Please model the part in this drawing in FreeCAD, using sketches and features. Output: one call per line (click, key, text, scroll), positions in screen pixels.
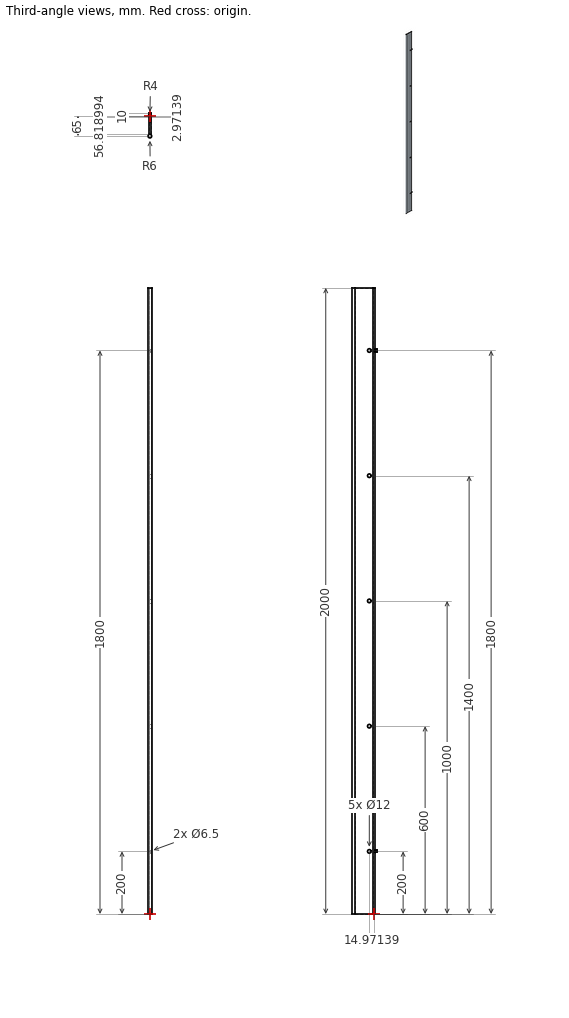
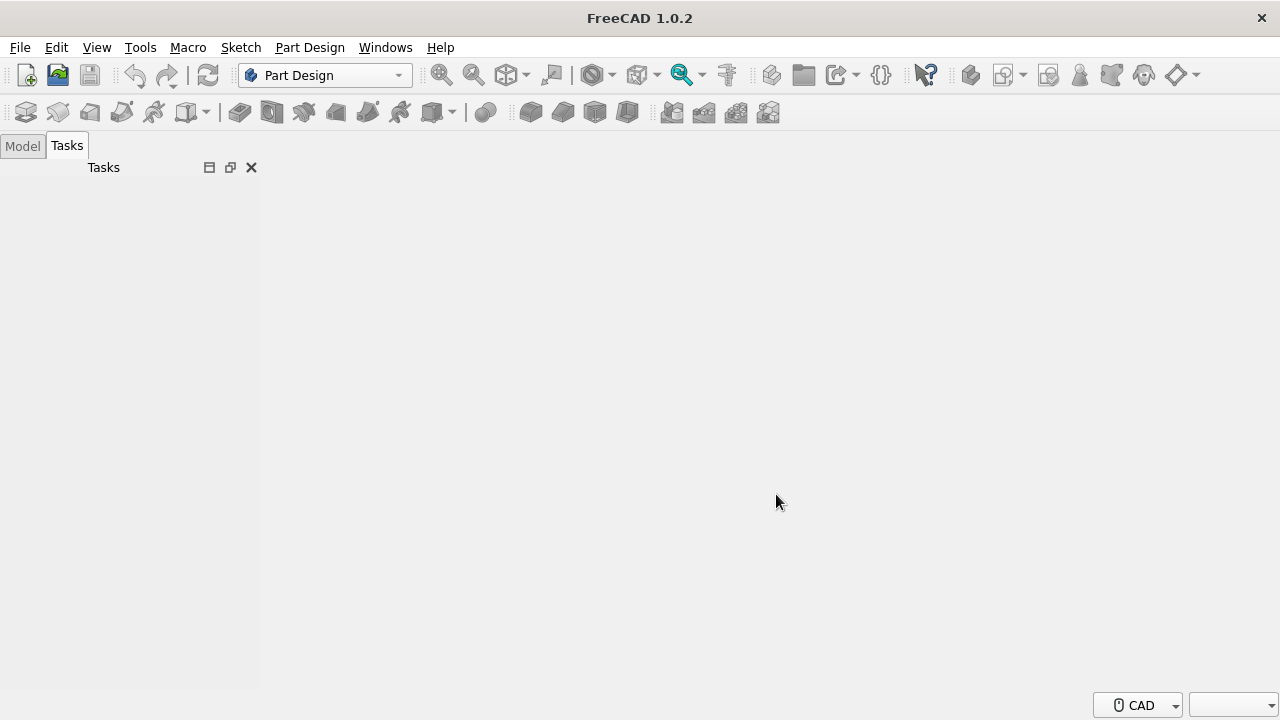
key(ctrl+n)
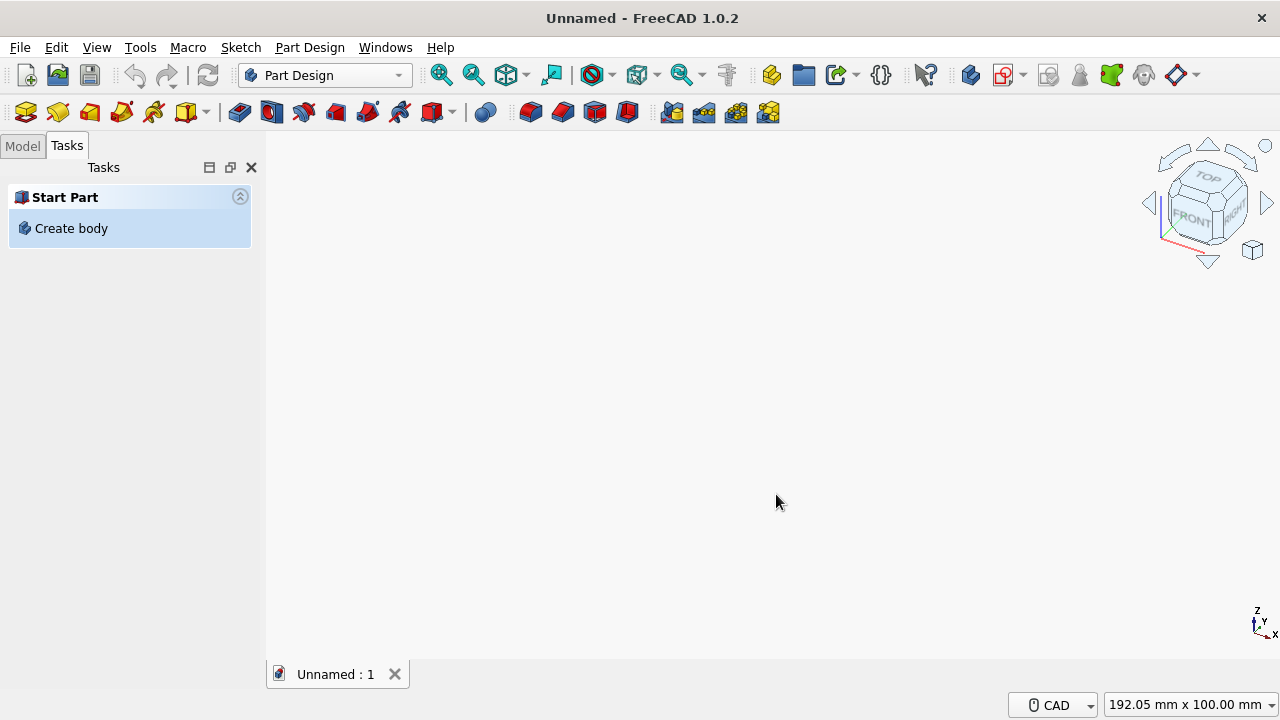
click(1004, 76)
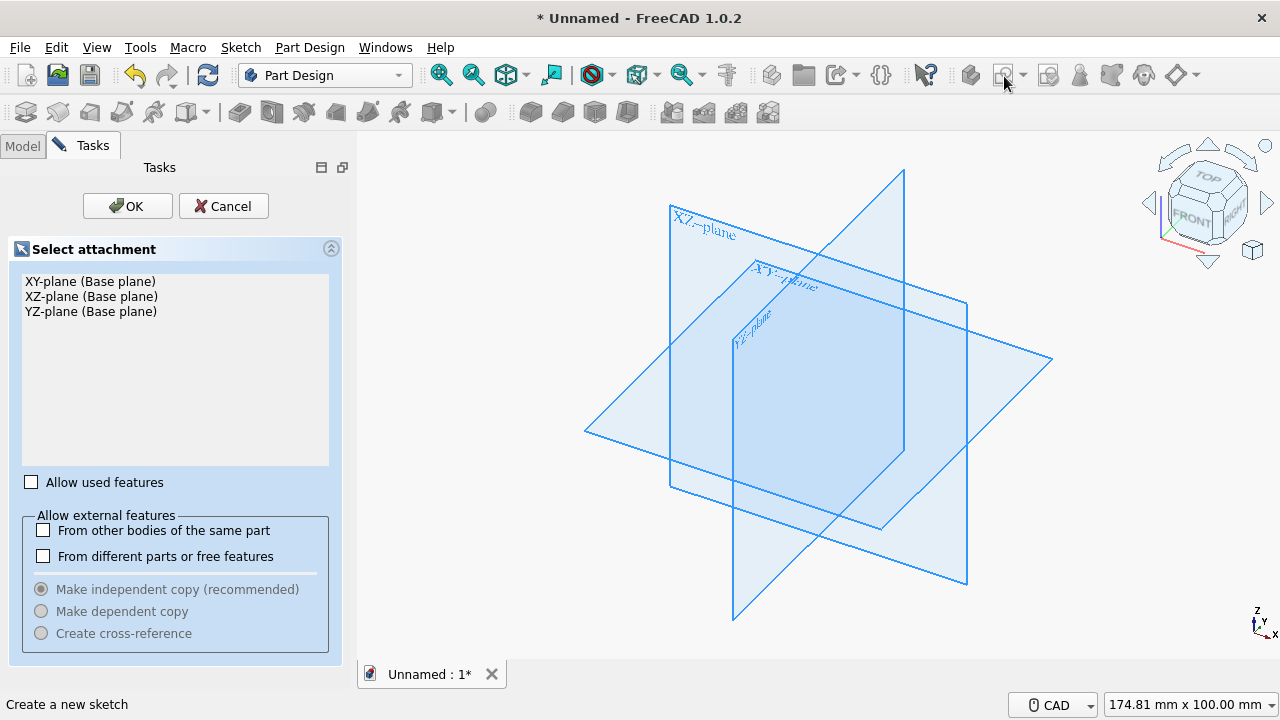
click(82, 282)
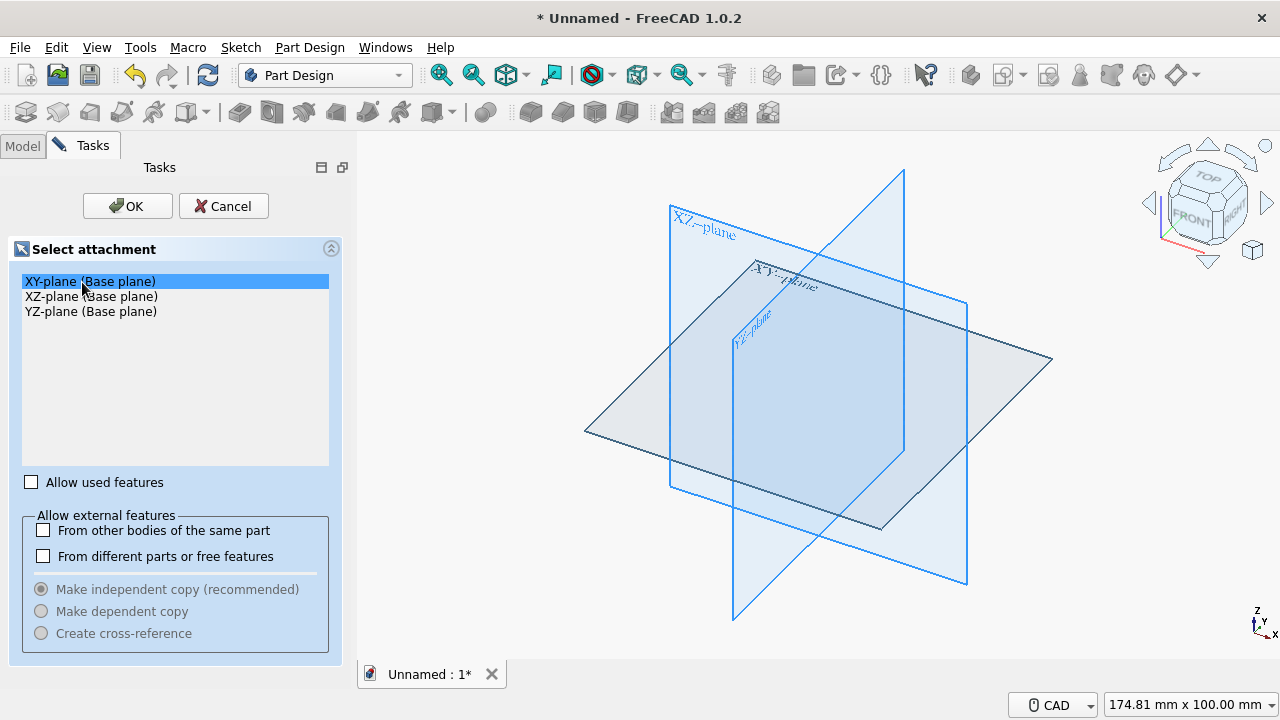
click(128, 206)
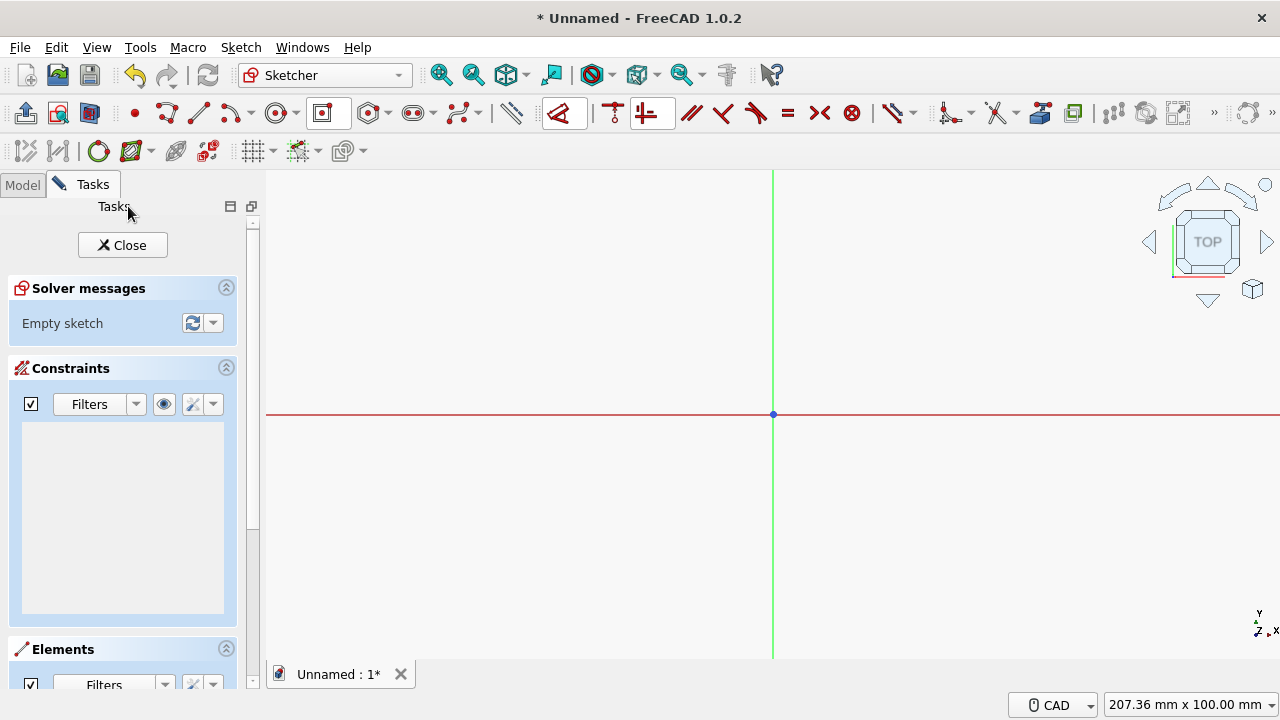
scroll(566, 198, down, 2)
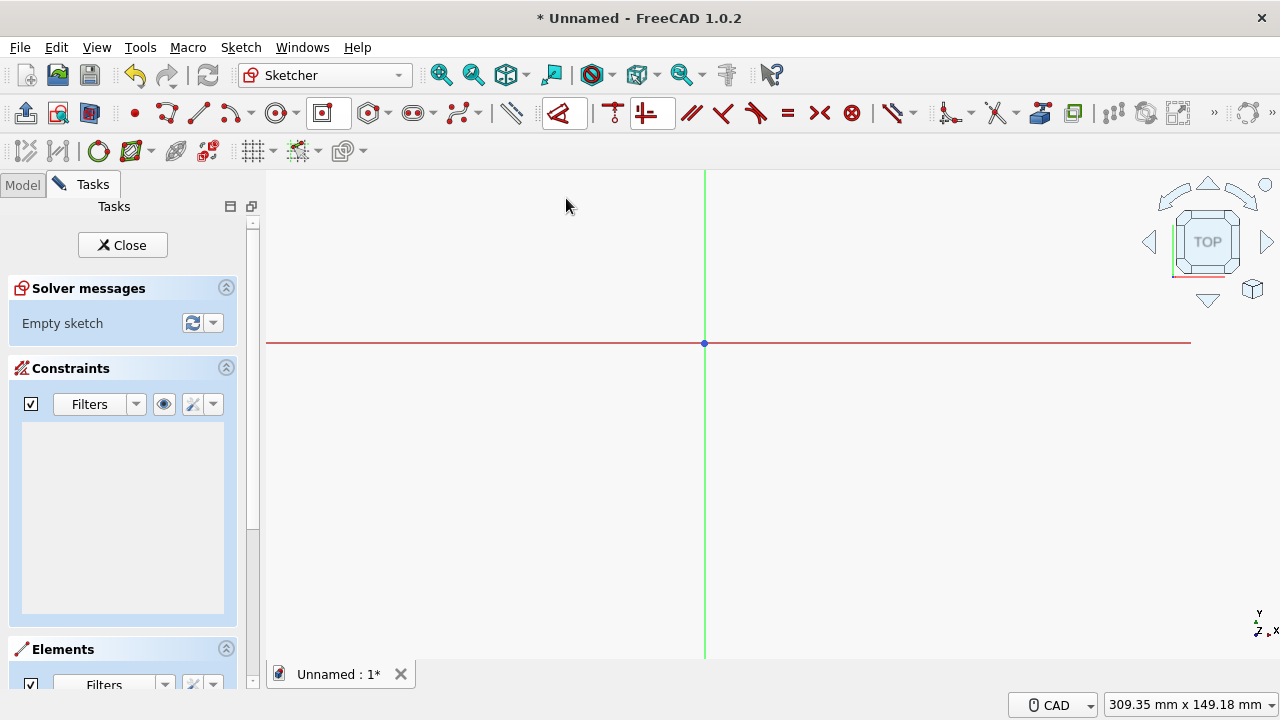
key(g)
key(l)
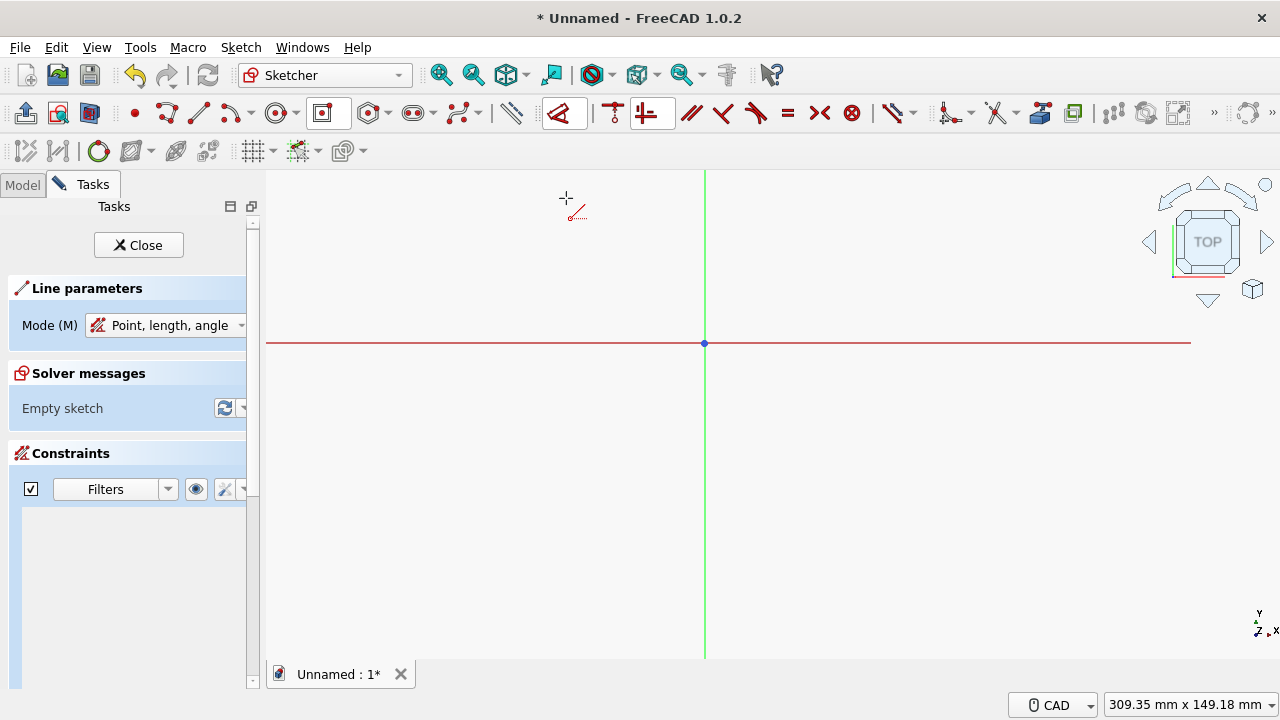
scroll(696, 353, up, 3)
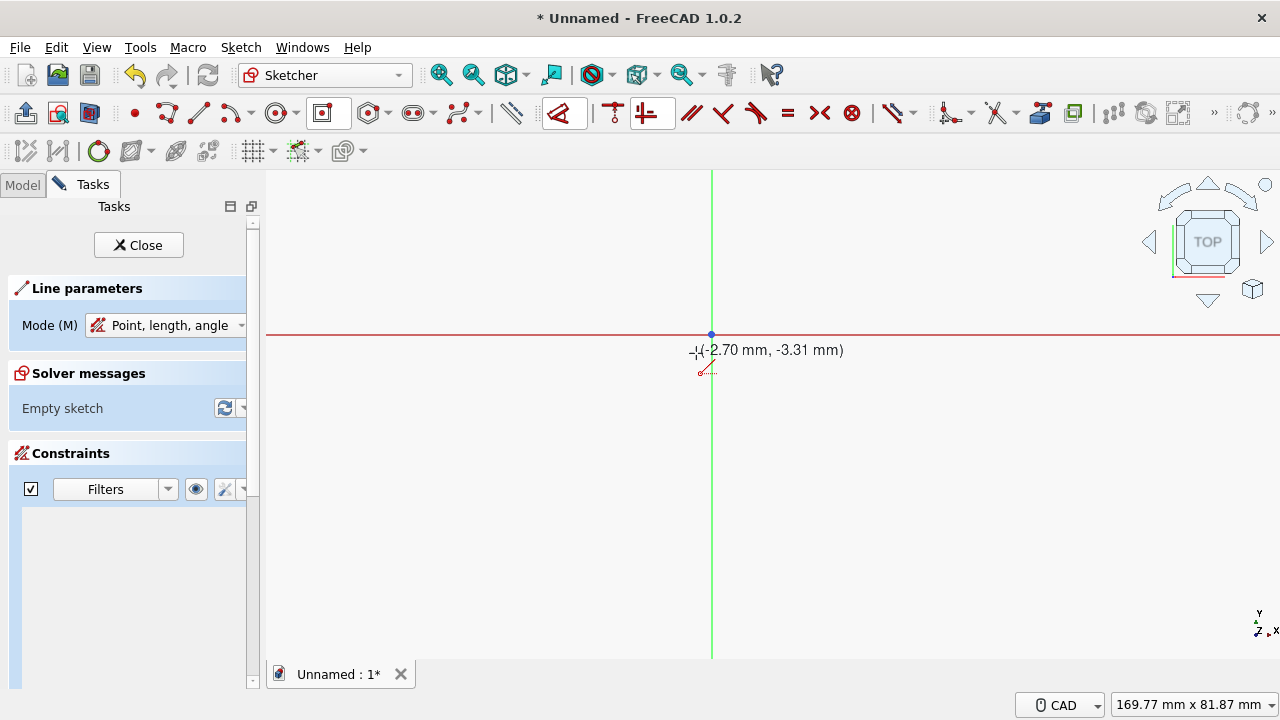
click(695, 352)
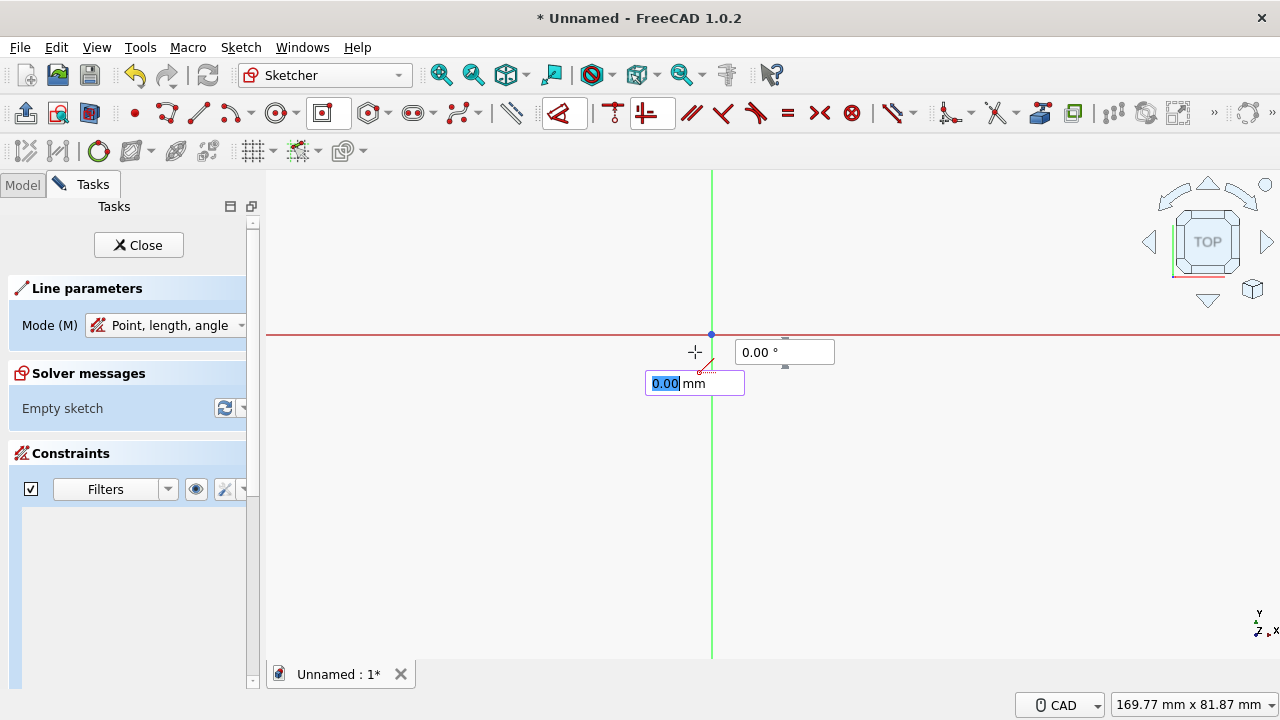
scroll(690, 198, down, 2)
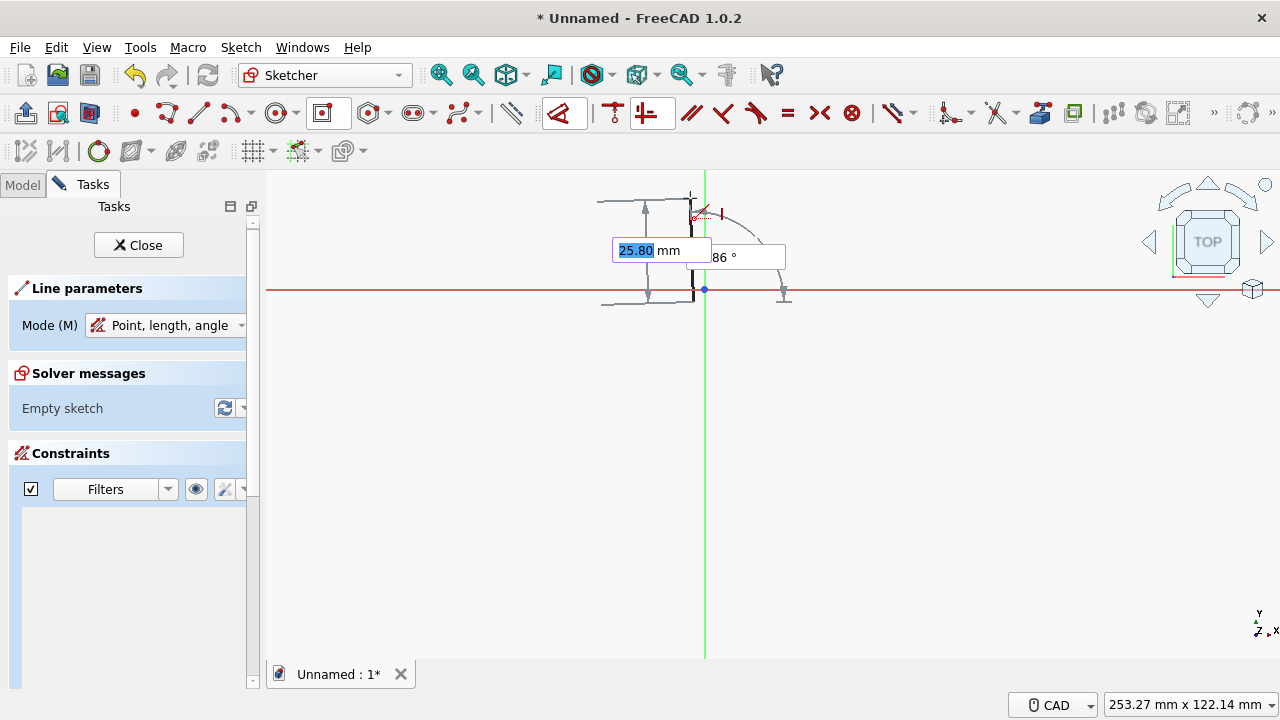
scroll(694, 529, up, 2)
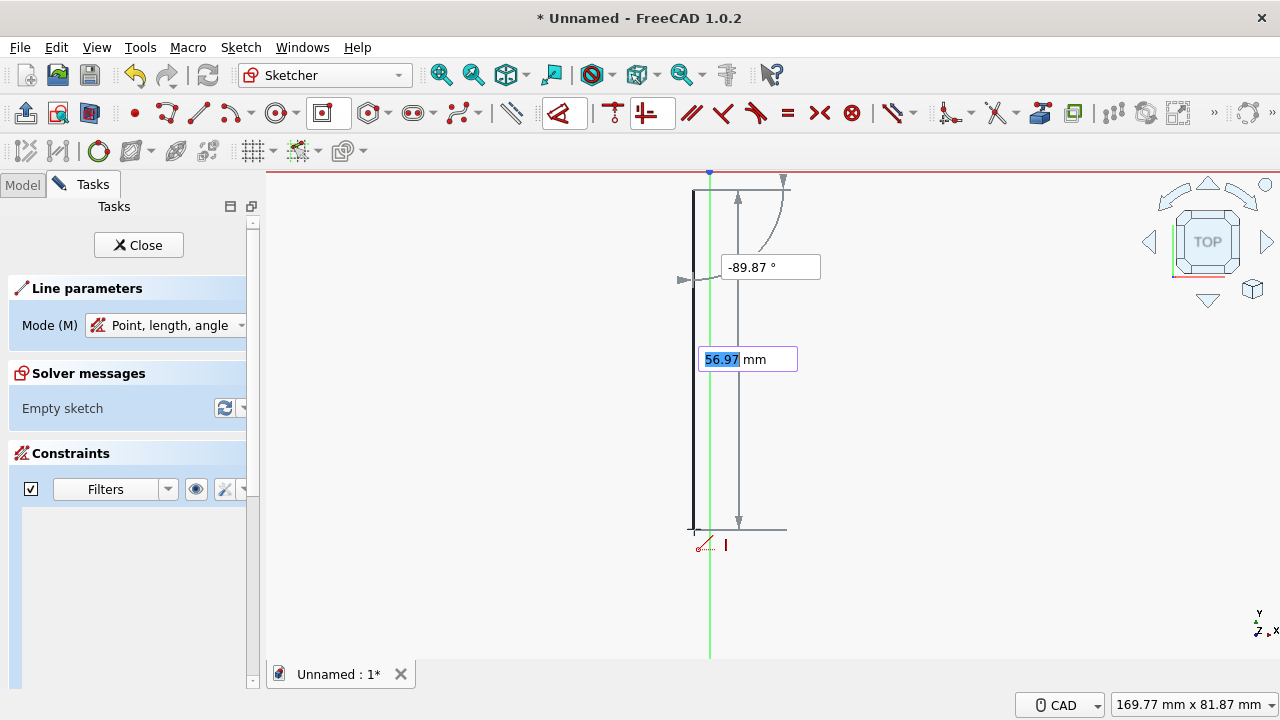
click(693, 528)